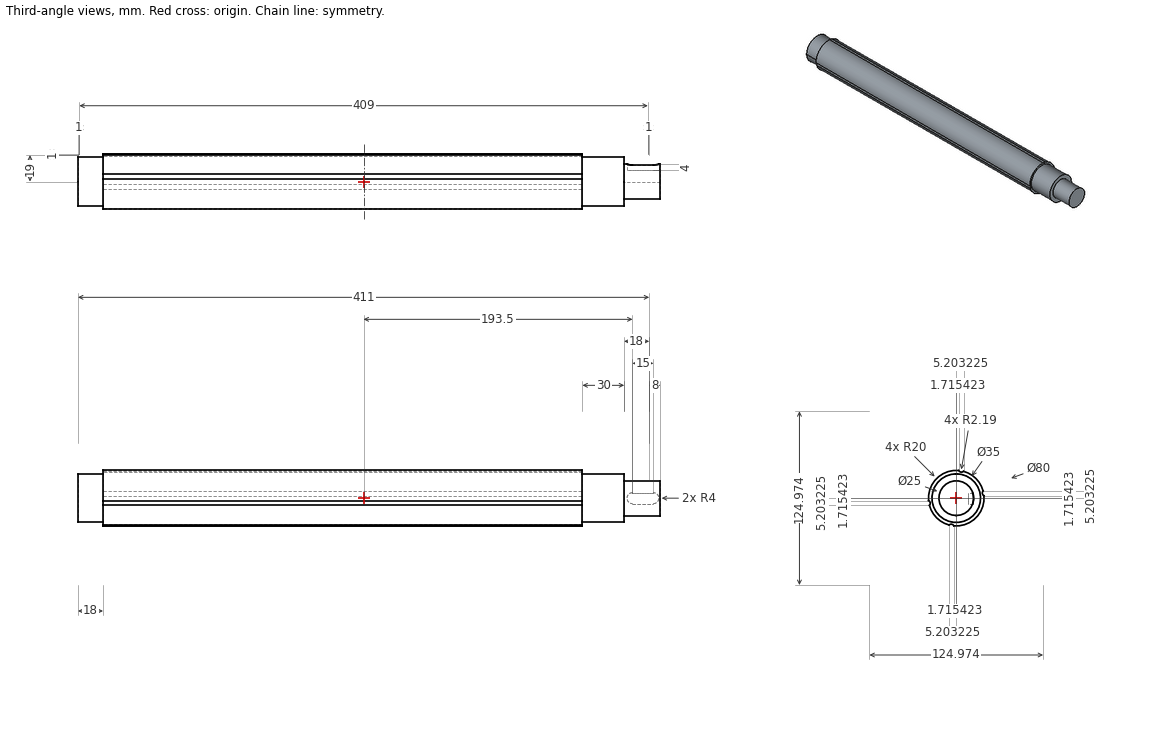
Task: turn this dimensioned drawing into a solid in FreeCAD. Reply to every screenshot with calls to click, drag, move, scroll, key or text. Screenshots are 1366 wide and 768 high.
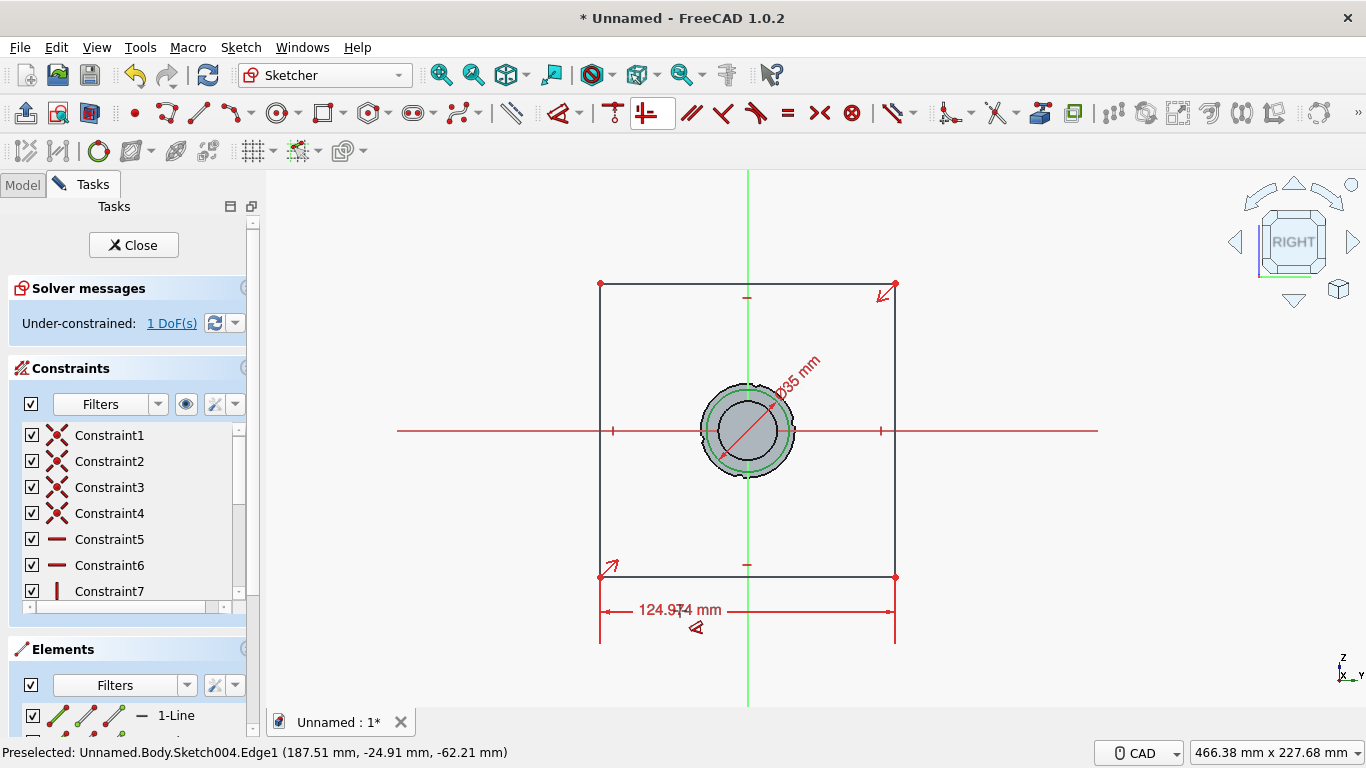
click(895, 489)
click(929, 363)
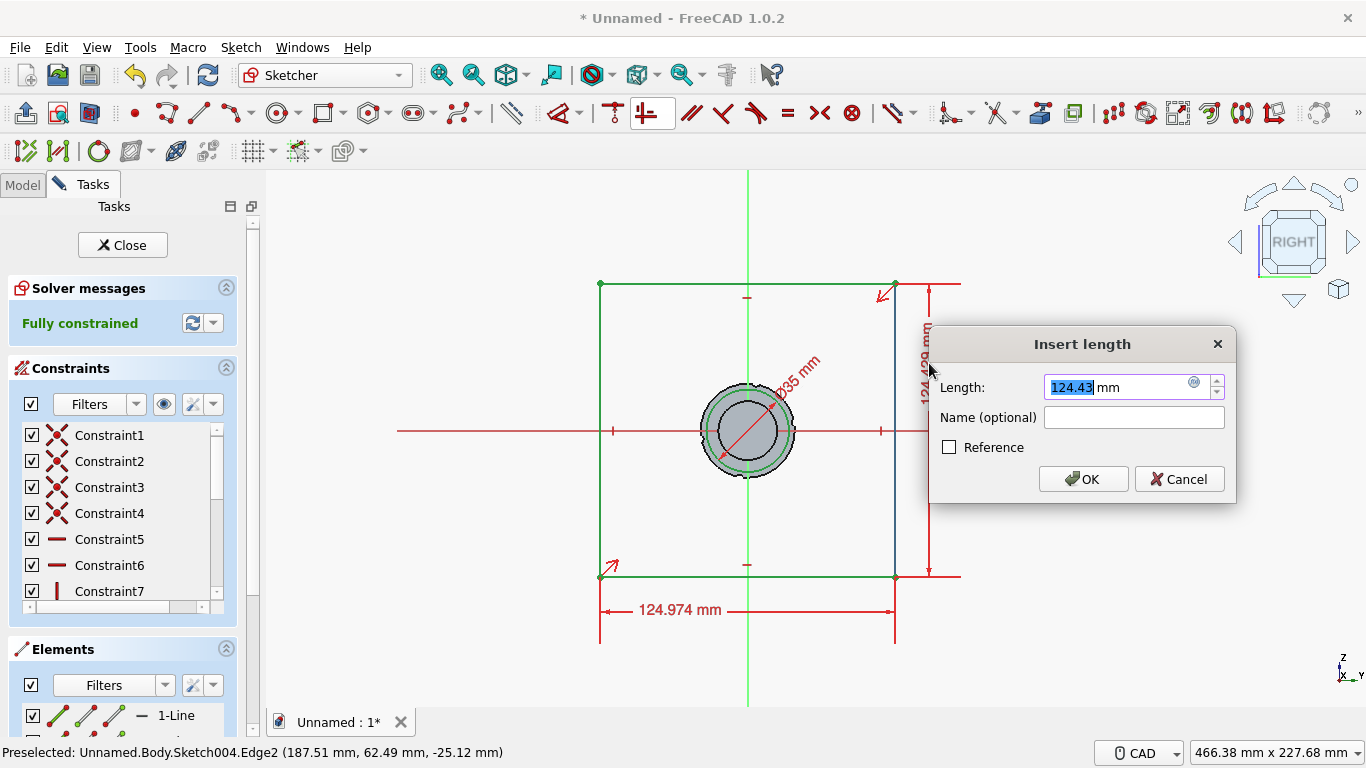
text(124.974)
key(Return)
key(Escape)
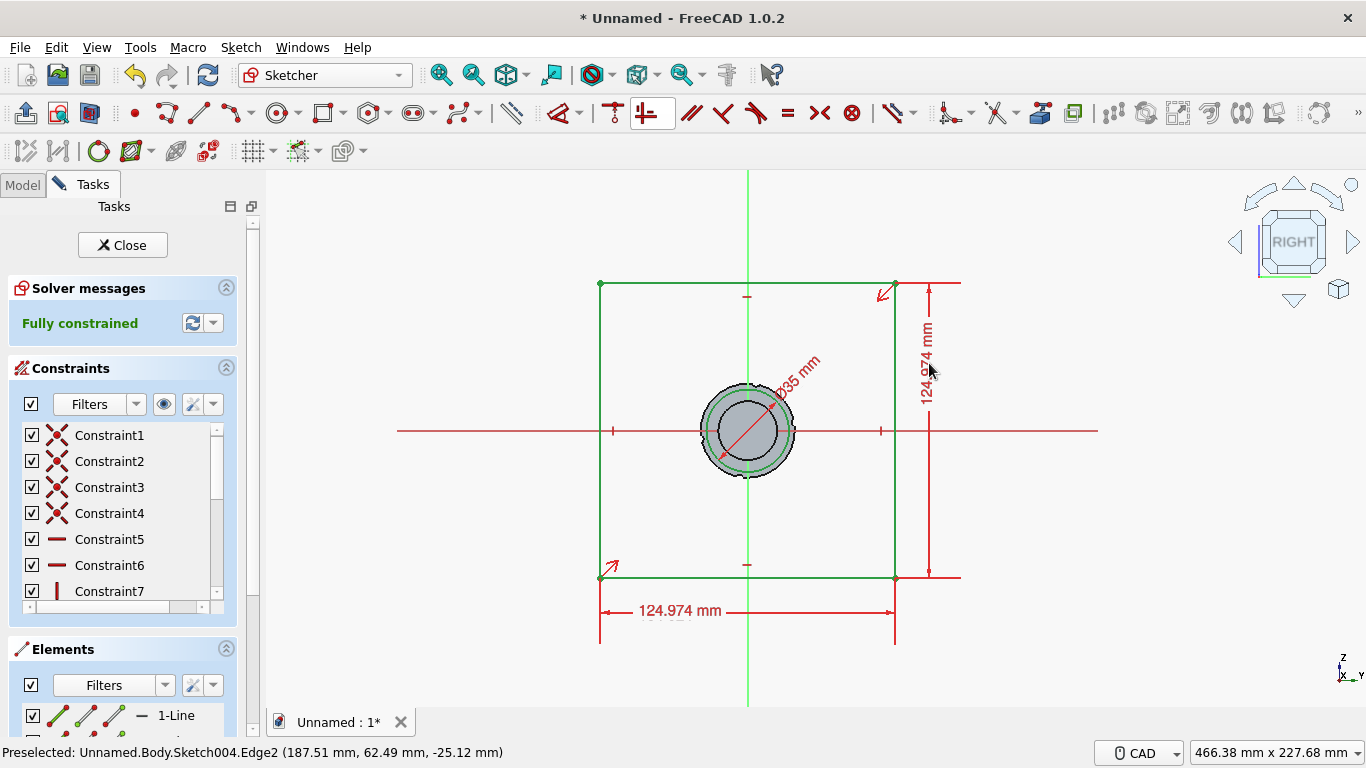
click(123, 245)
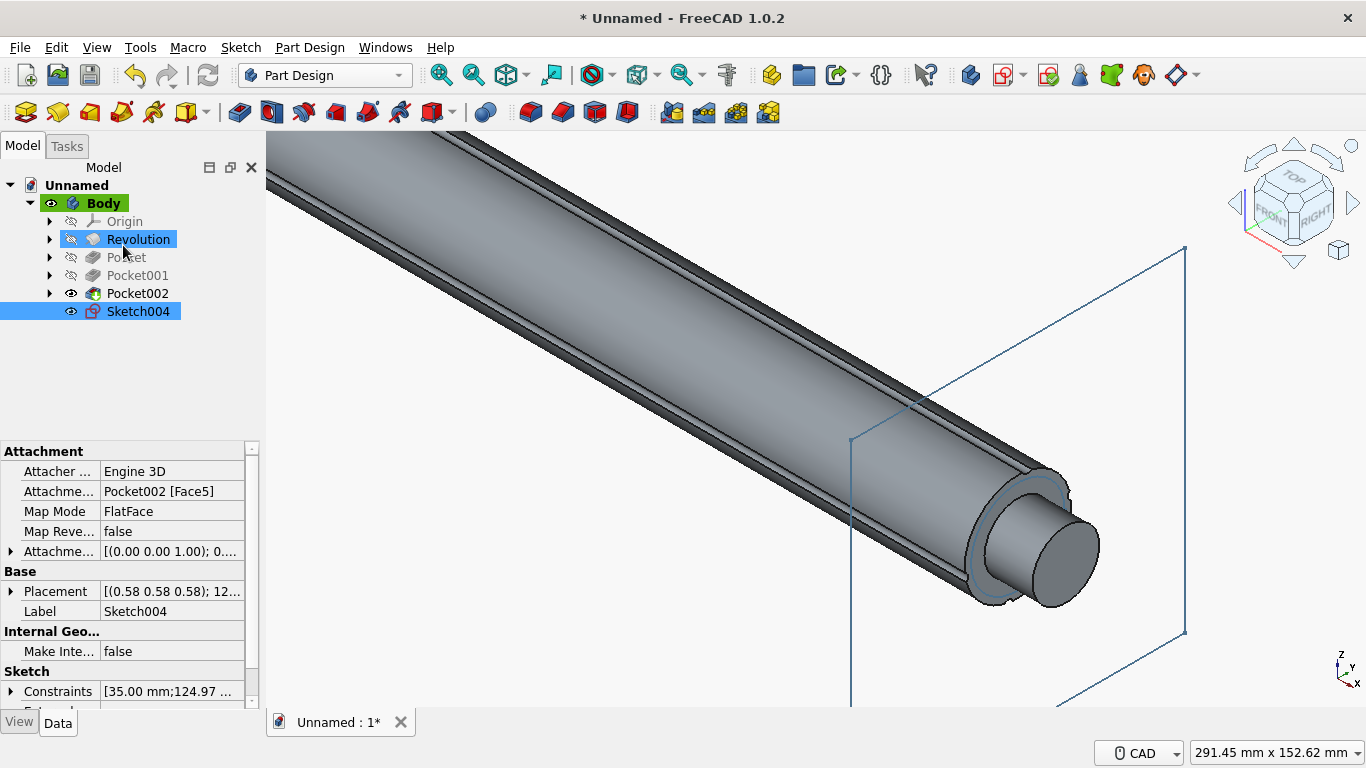
click(240, 112)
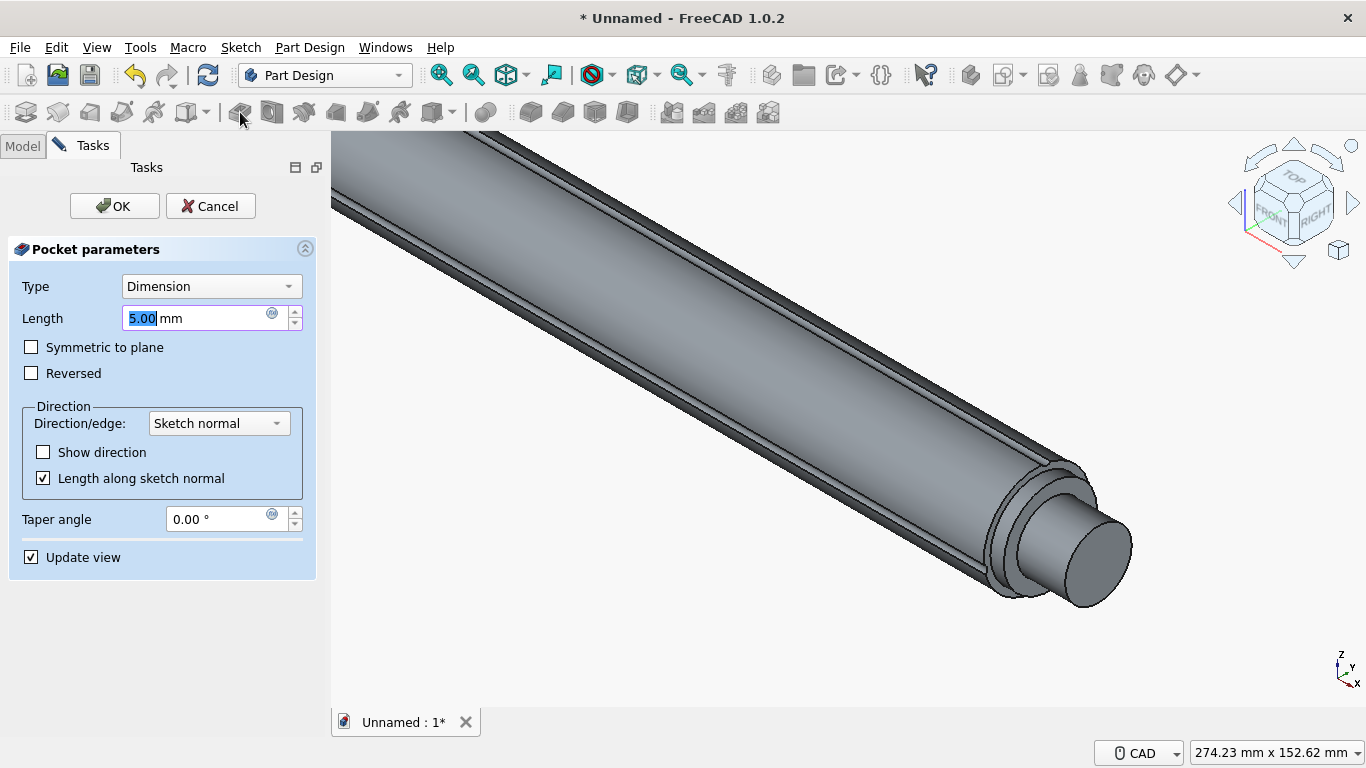
text(30)
key(Tab)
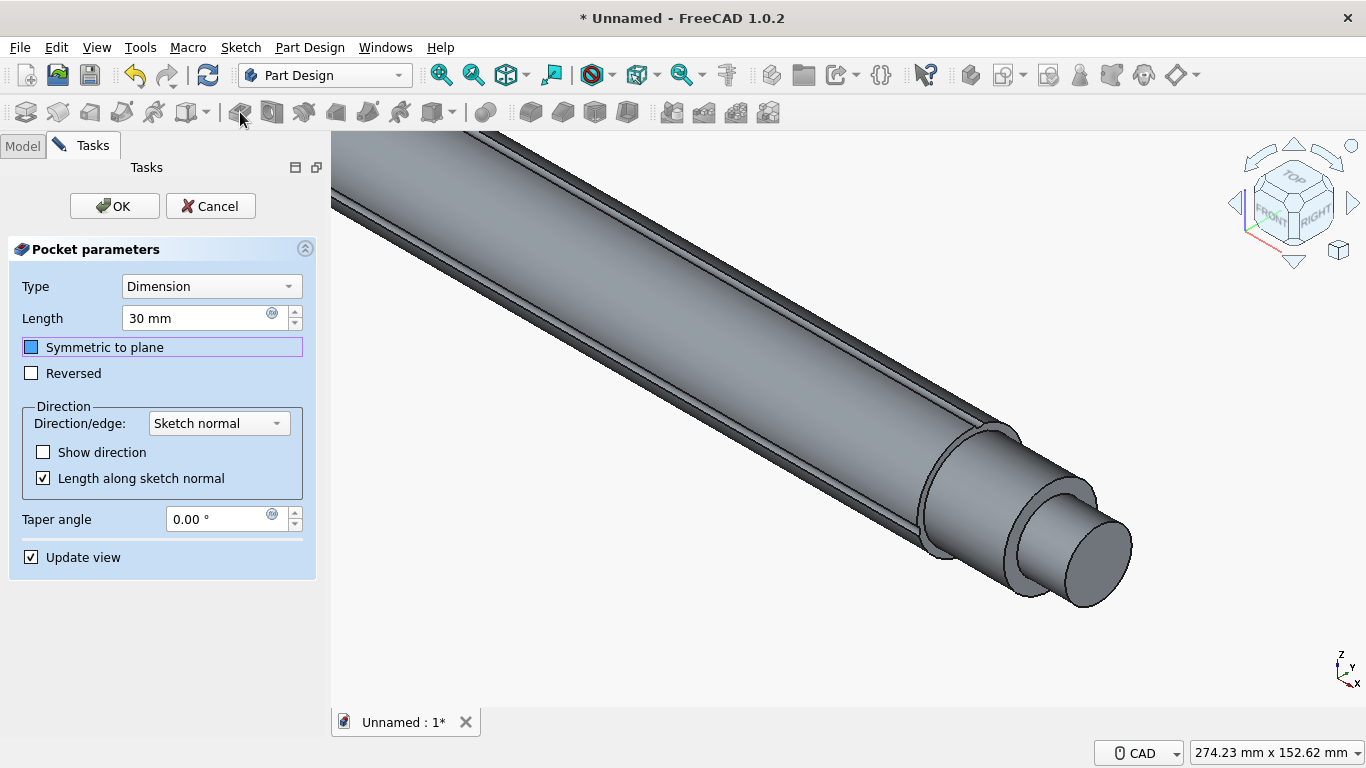
click(115, 206)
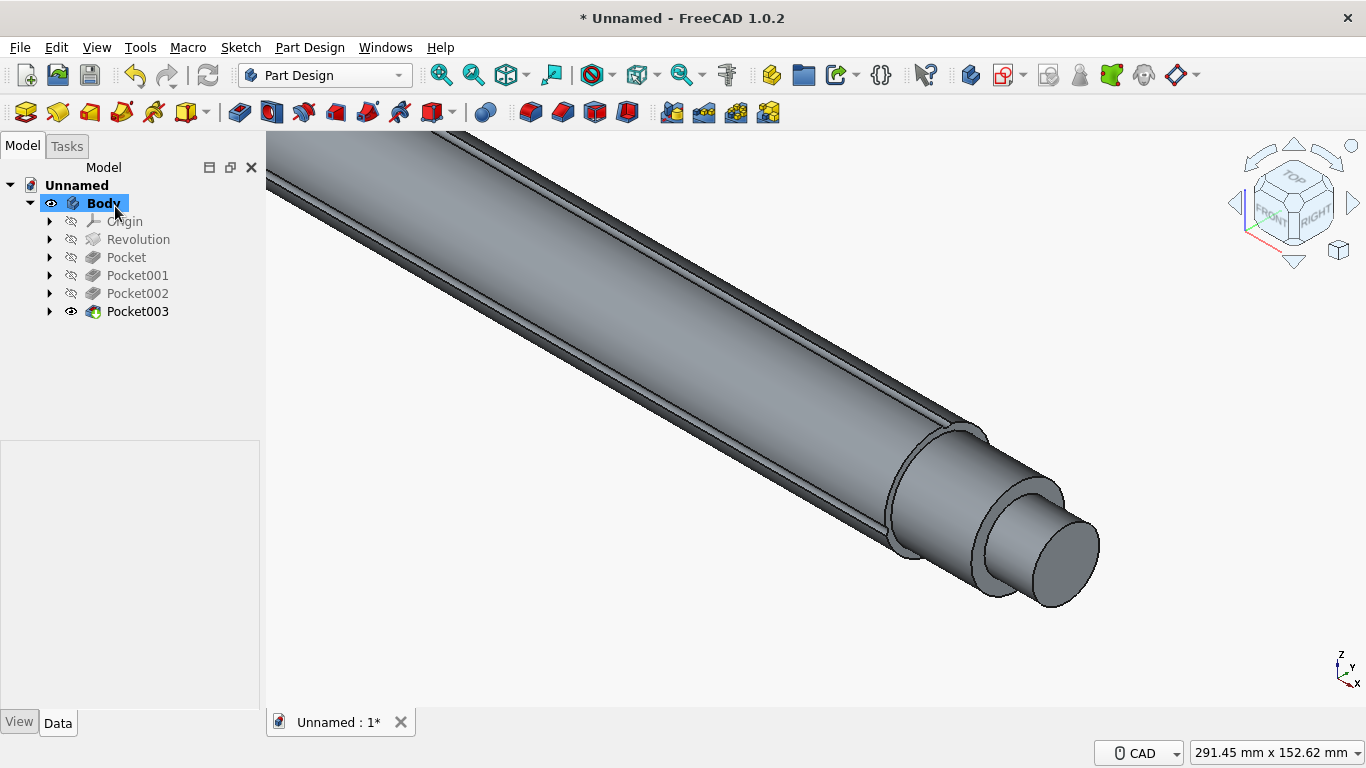
key(v)
key(f)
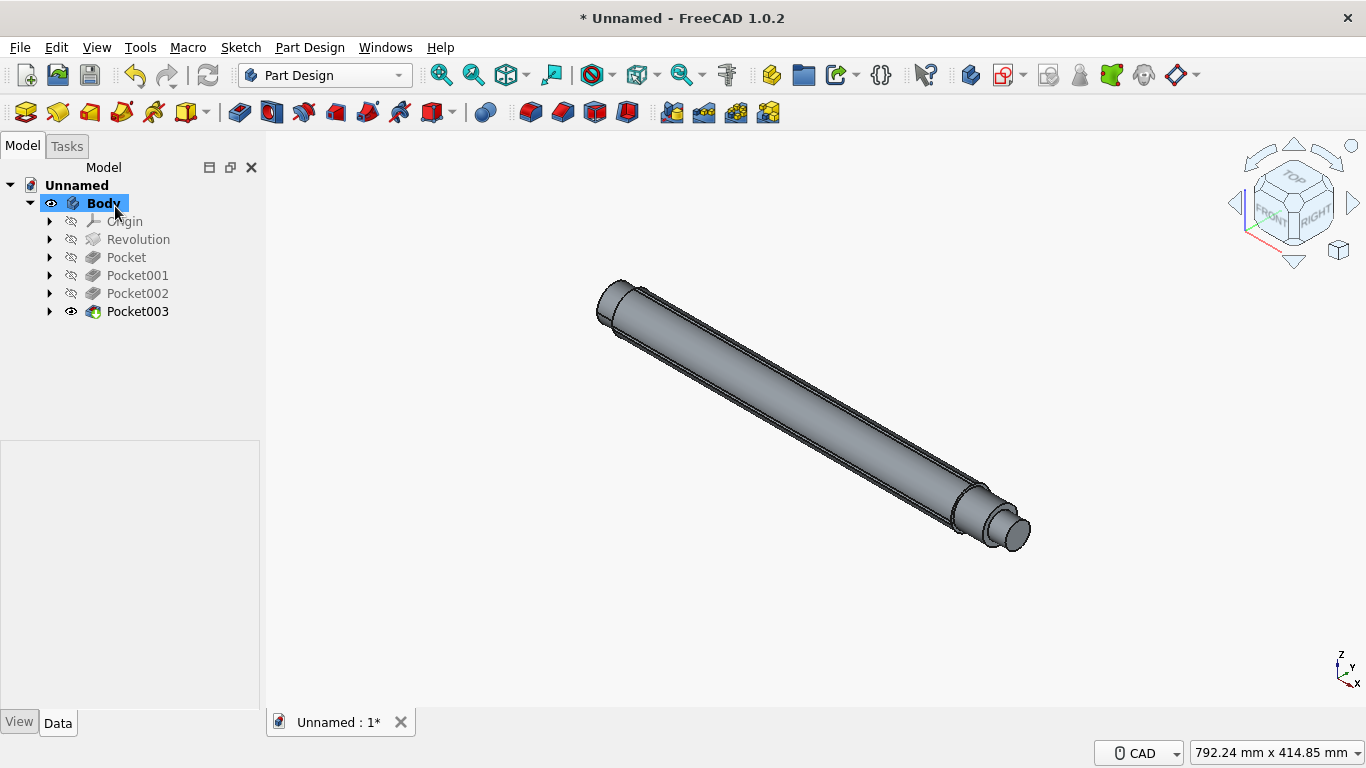
click(50, 221)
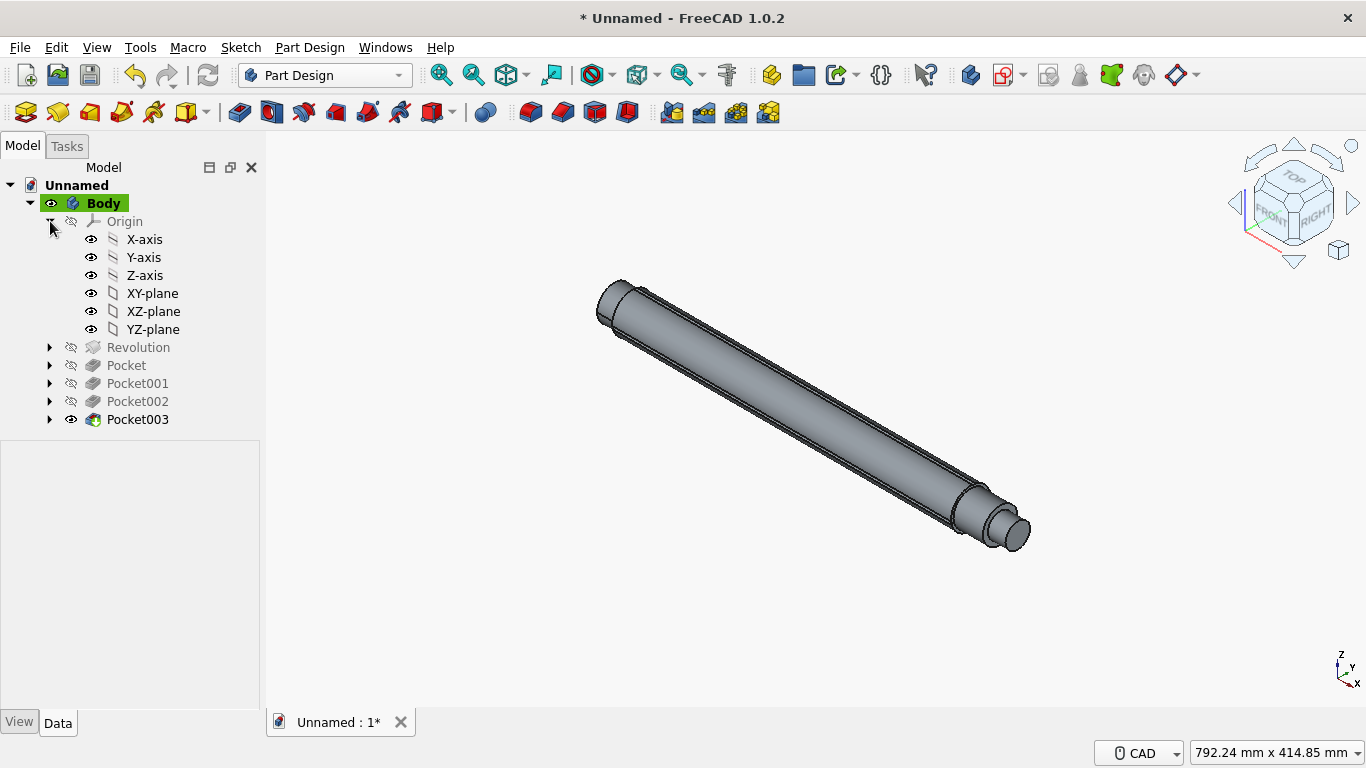
click(136, 329)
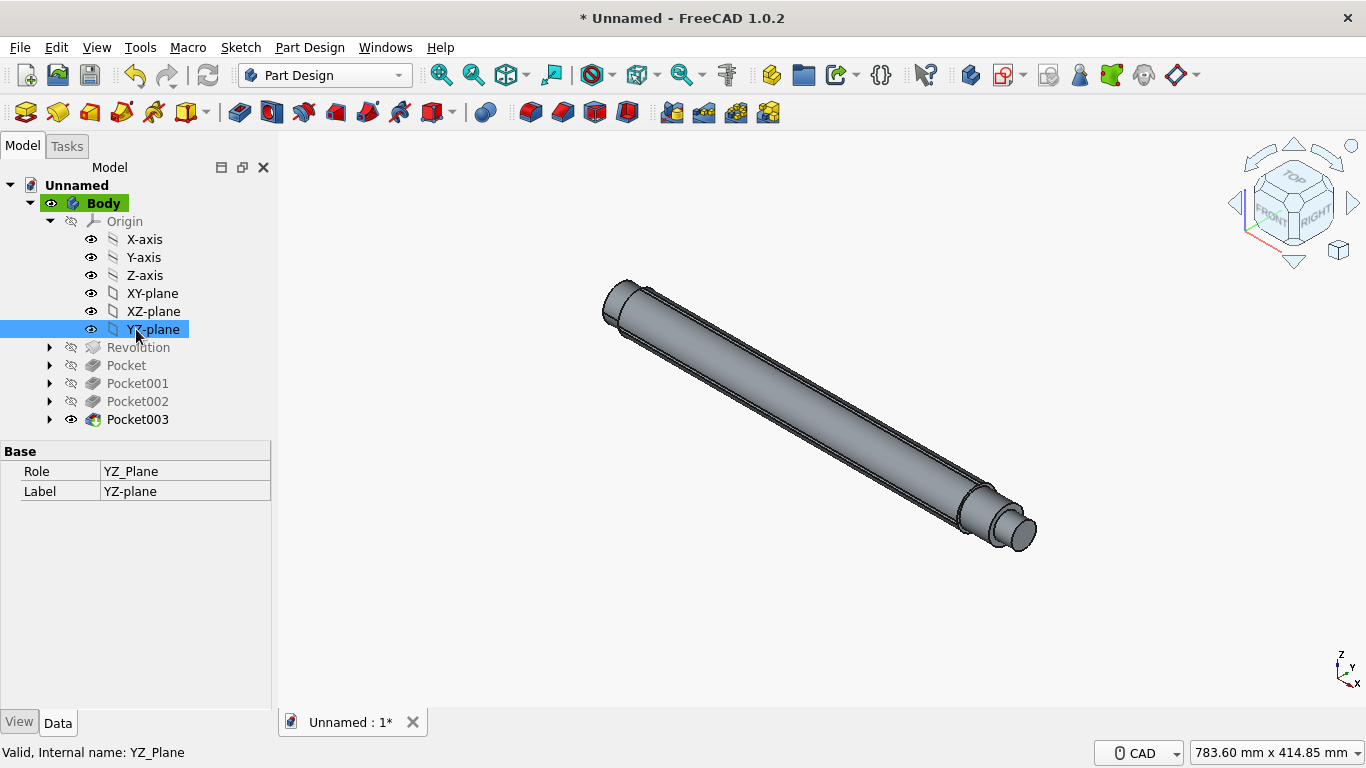
click(1176, 76)